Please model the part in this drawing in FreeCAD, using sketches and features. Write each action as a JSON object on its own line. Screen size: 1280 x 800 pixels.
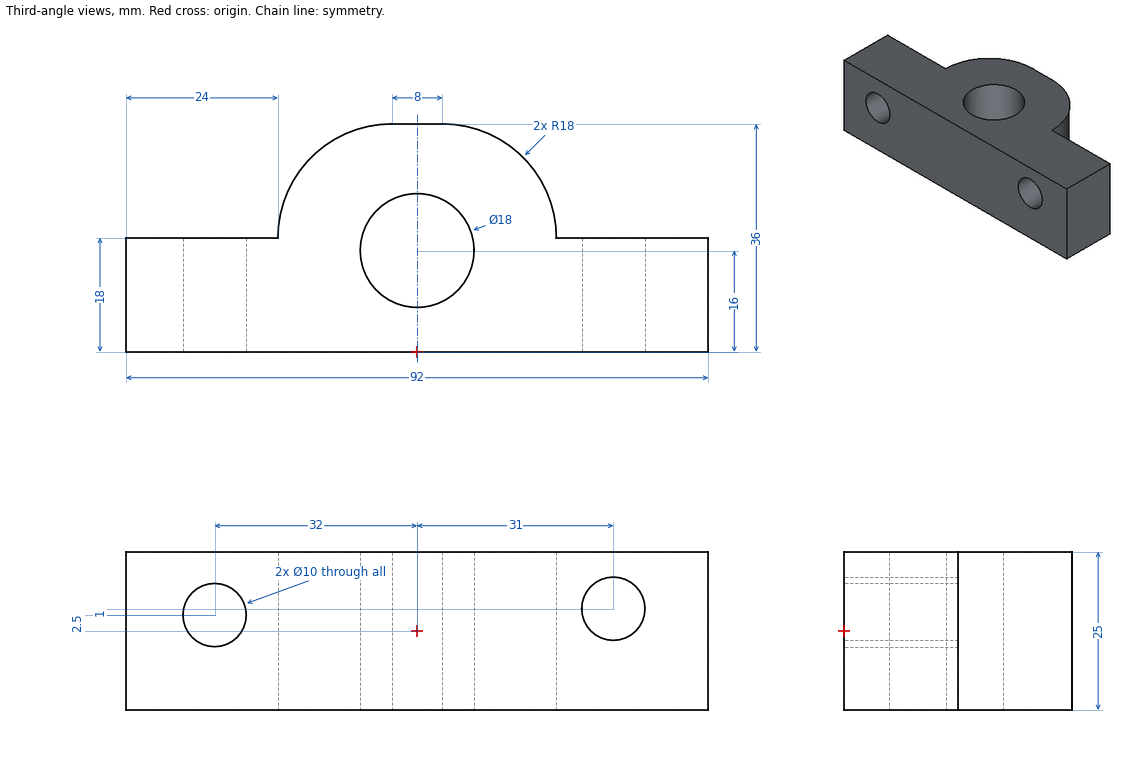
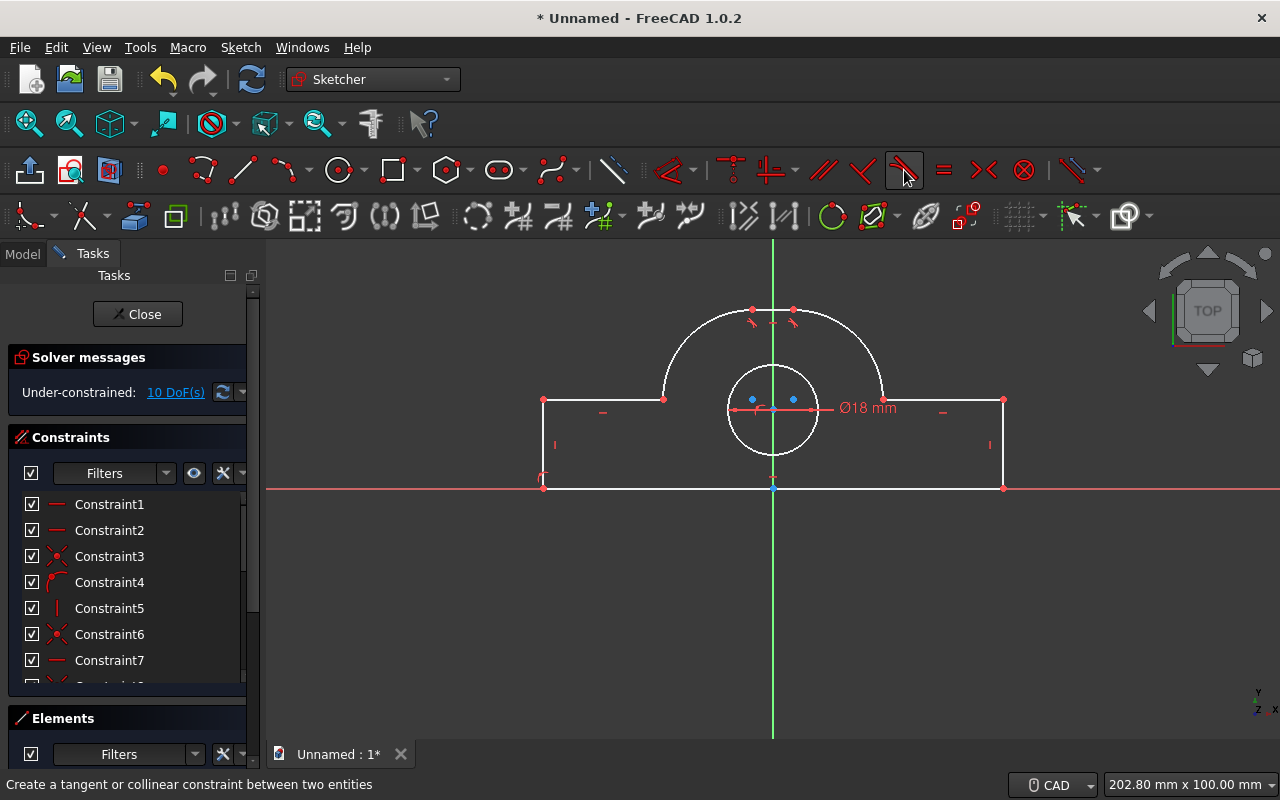
{"action": "left_click", "coordinate": [712, 320]}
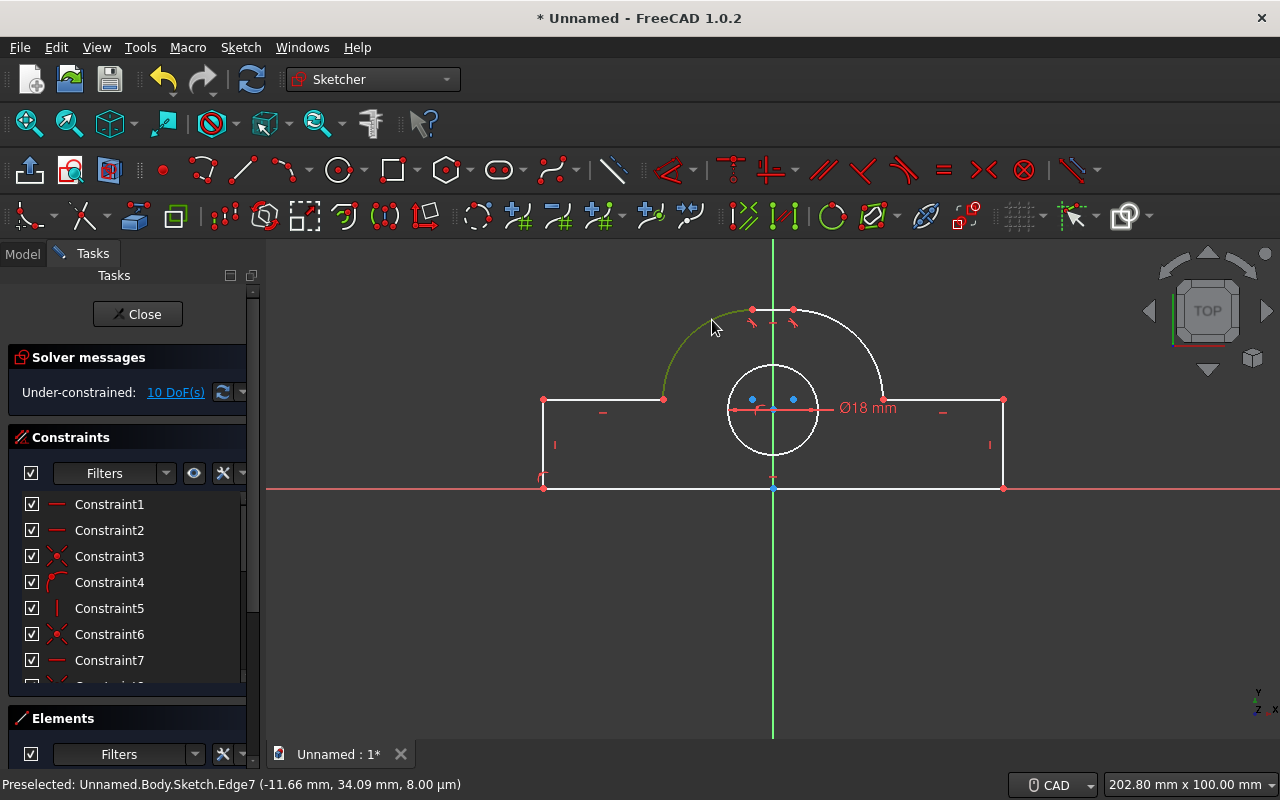
{"action": "left_click", "coordinate": [873, 359]}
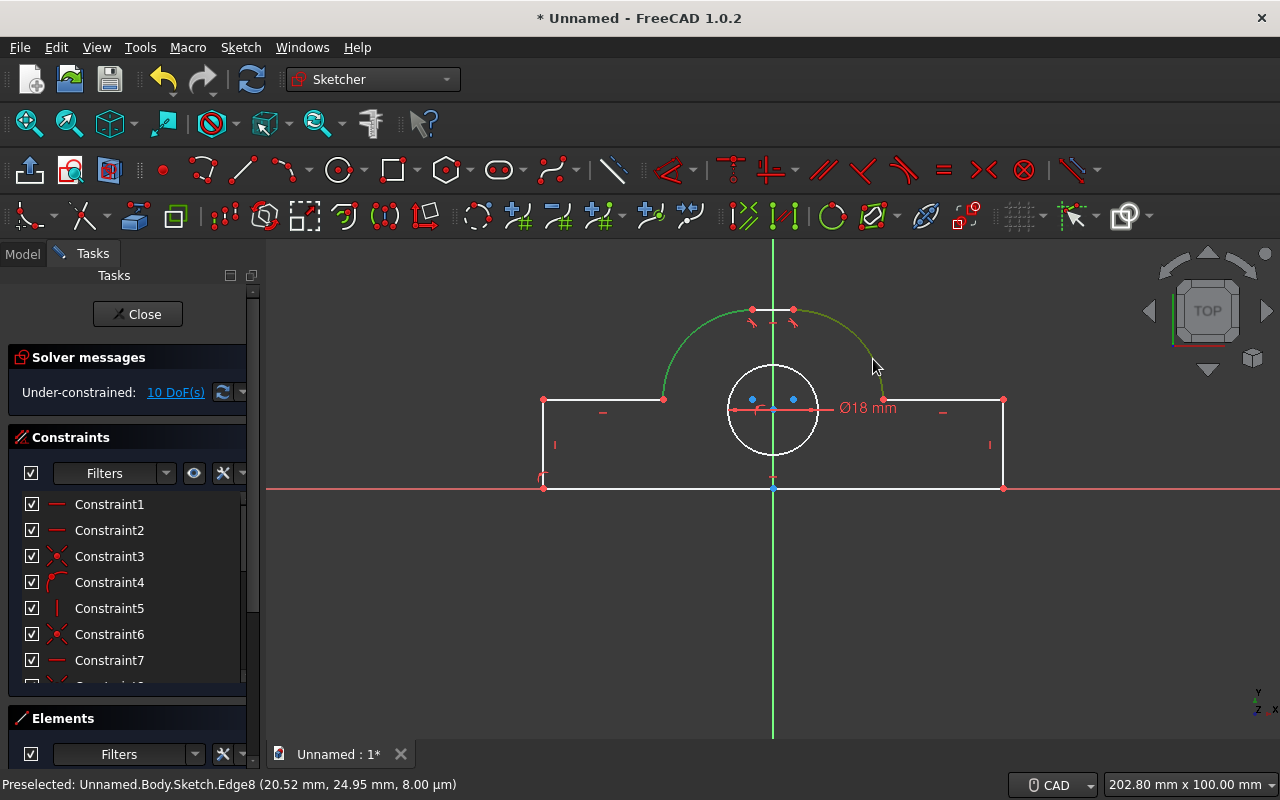
{"action": "key", "text": "e"}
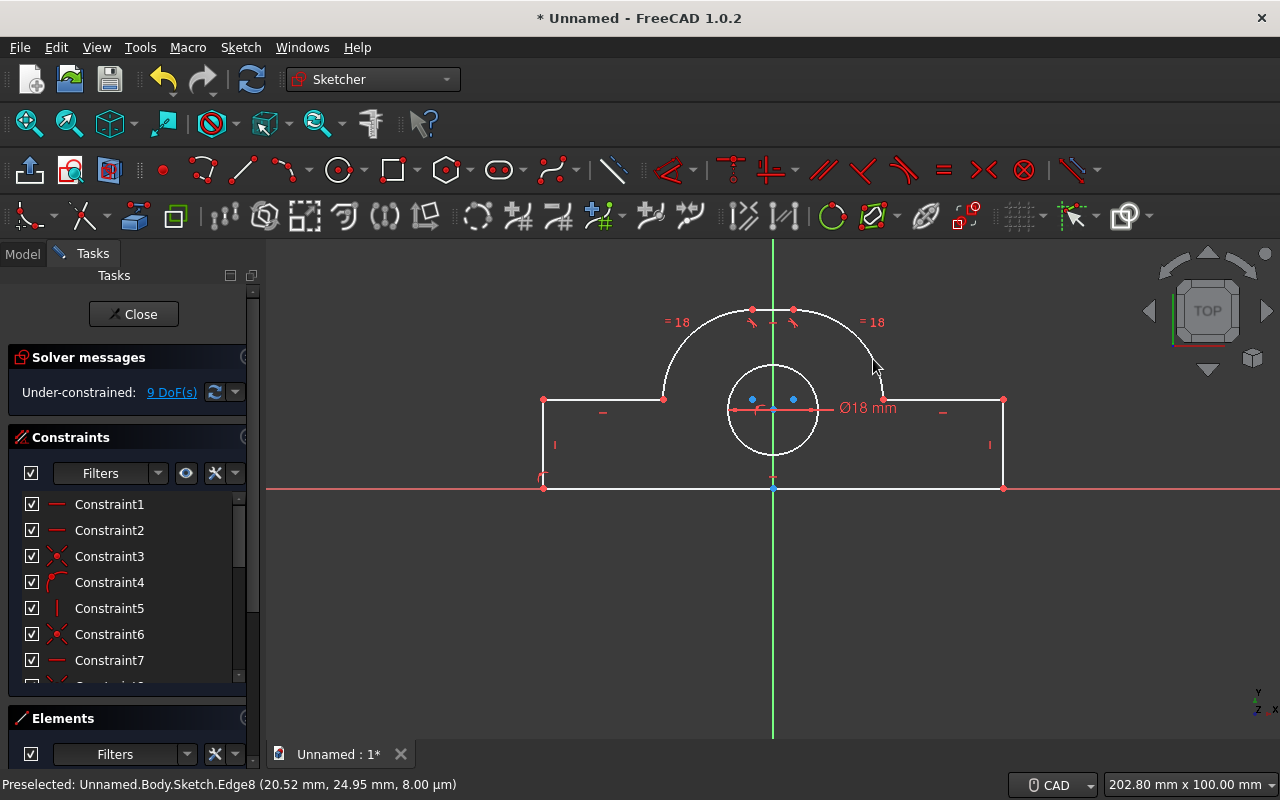
{"action": "left_click", "coordinate": [543, 400]}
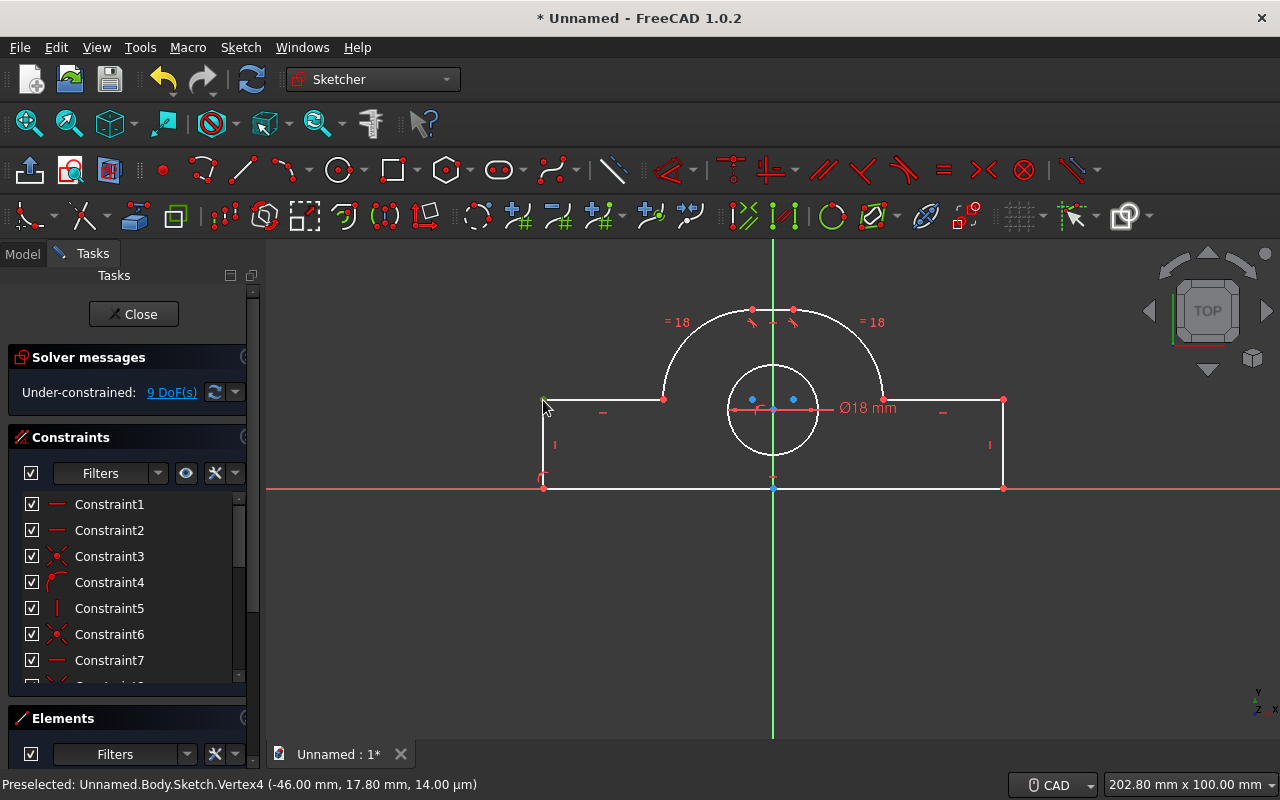
{"action": "left_click", "coordinate": [1003, 400]}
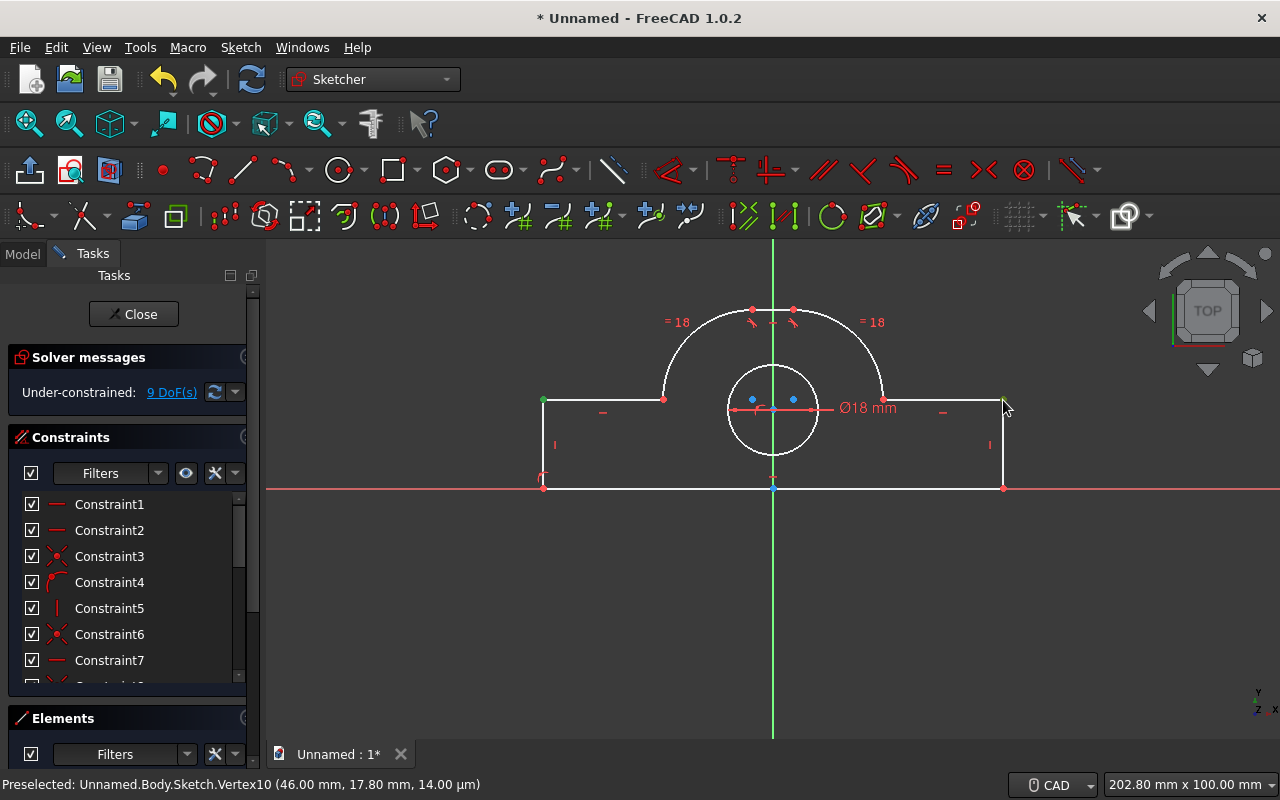
{"action": "left_click", "coordinate": [773, 679]}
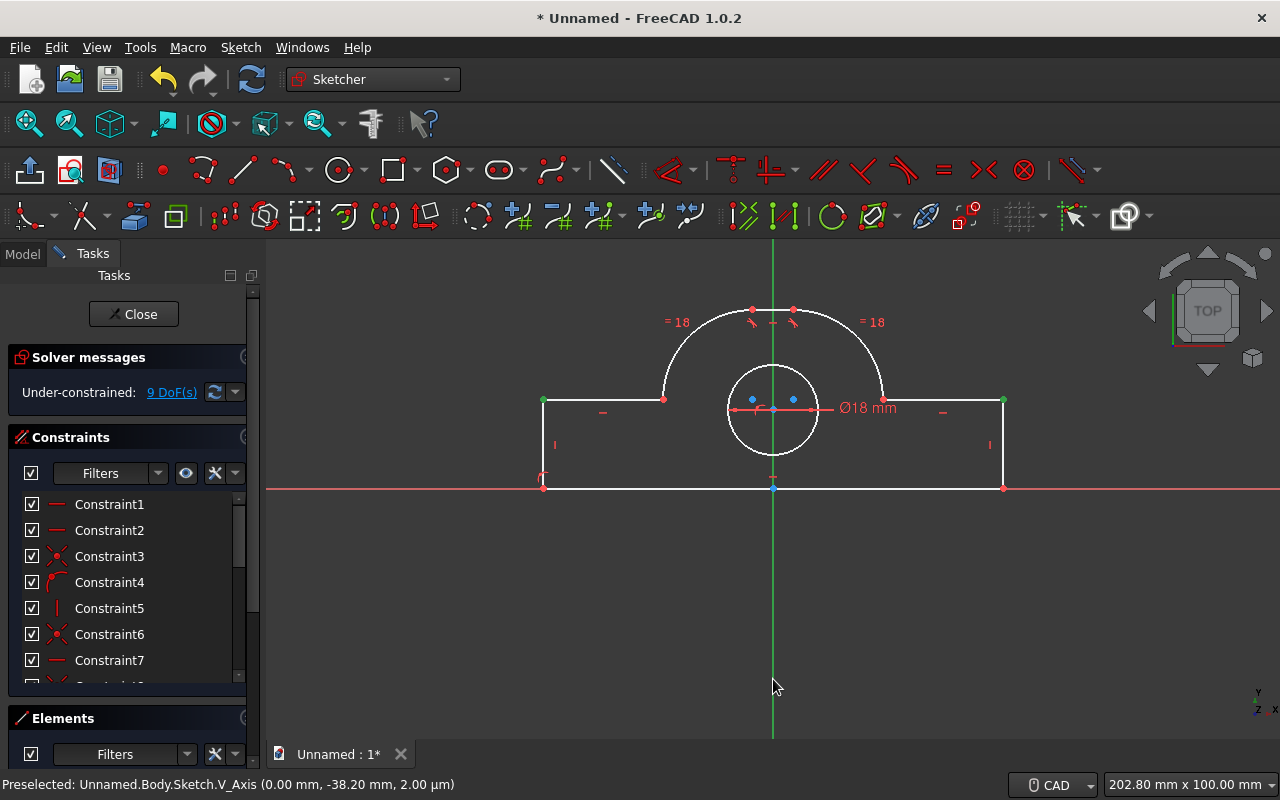
{"action": "left_click", "coordinate": [984, 170]}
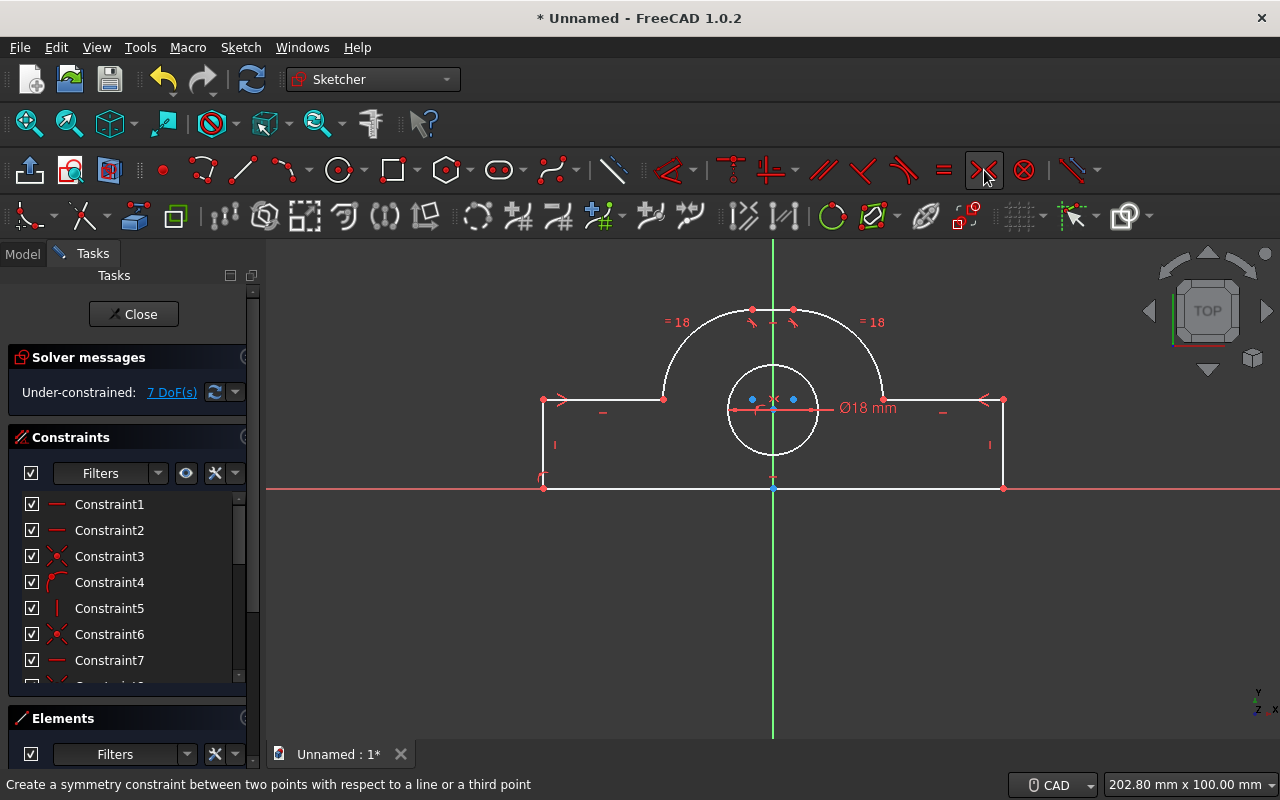
{"action": "left_click", "coordinate": [668, 170]}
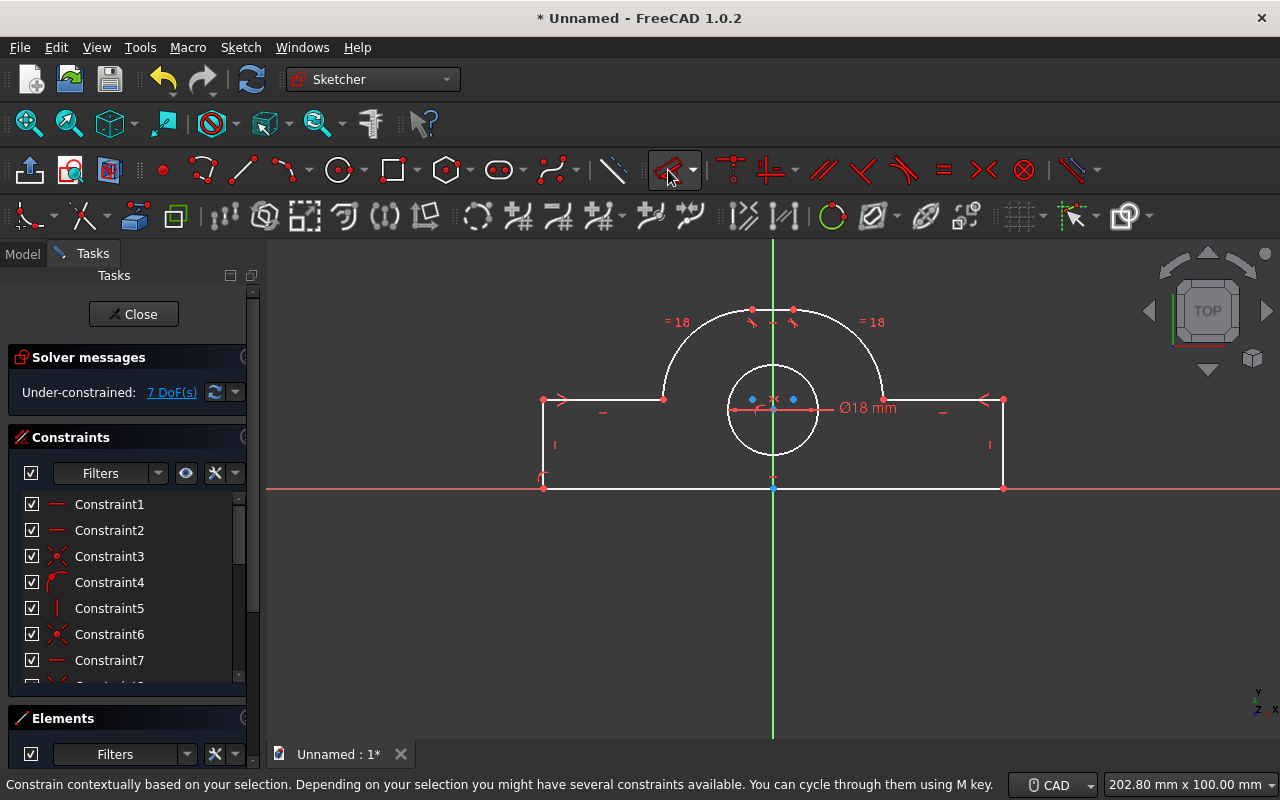
{"action": "left_click", "coordinate": [712, 320]}
{"action": "left_click", "coordinate": [697, 292]}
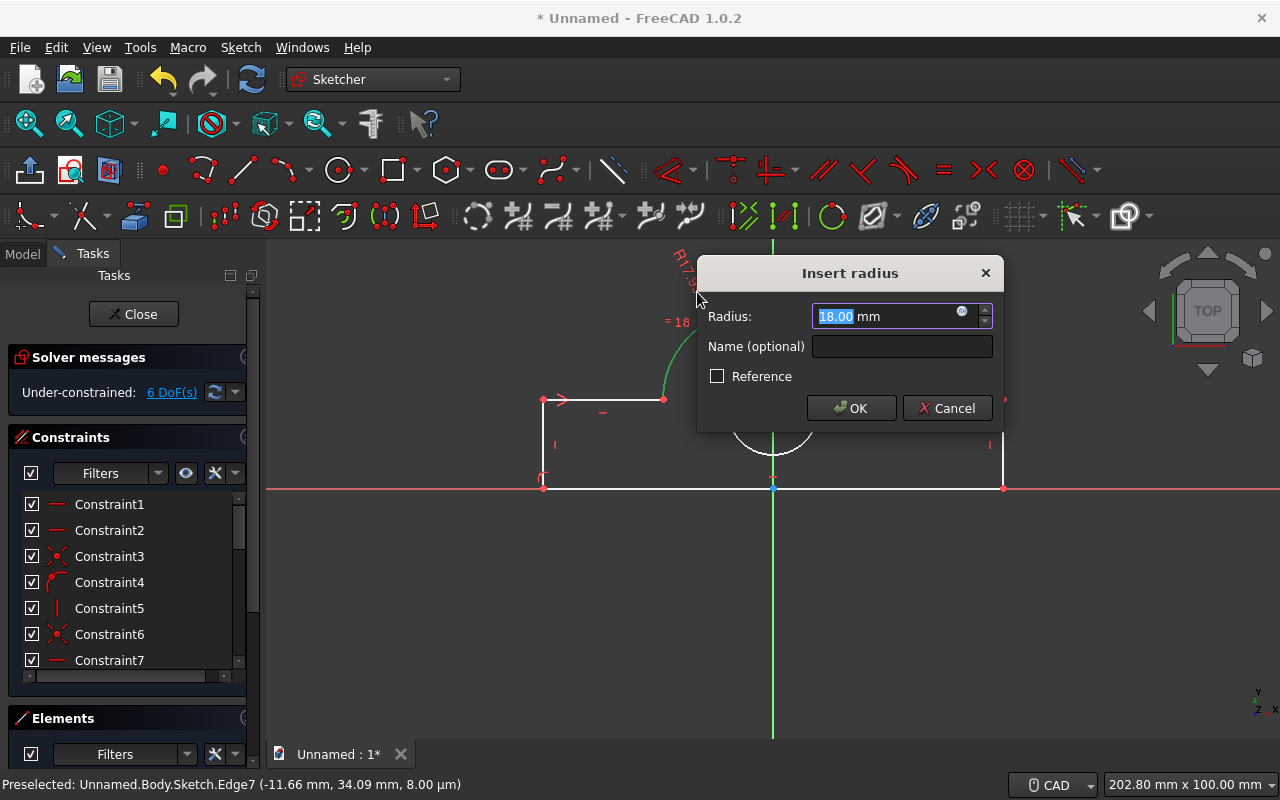
{"action": "type", "text": "18"}
{"action": "key", "text": "Return"}